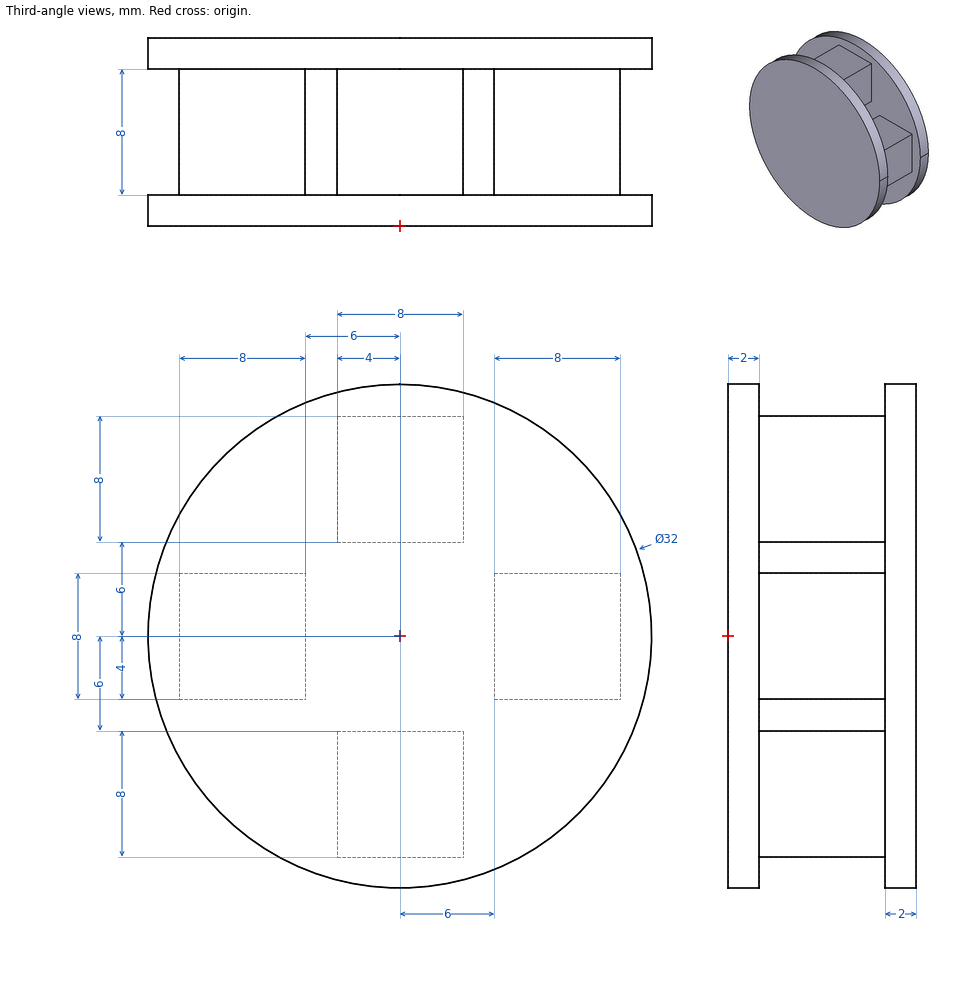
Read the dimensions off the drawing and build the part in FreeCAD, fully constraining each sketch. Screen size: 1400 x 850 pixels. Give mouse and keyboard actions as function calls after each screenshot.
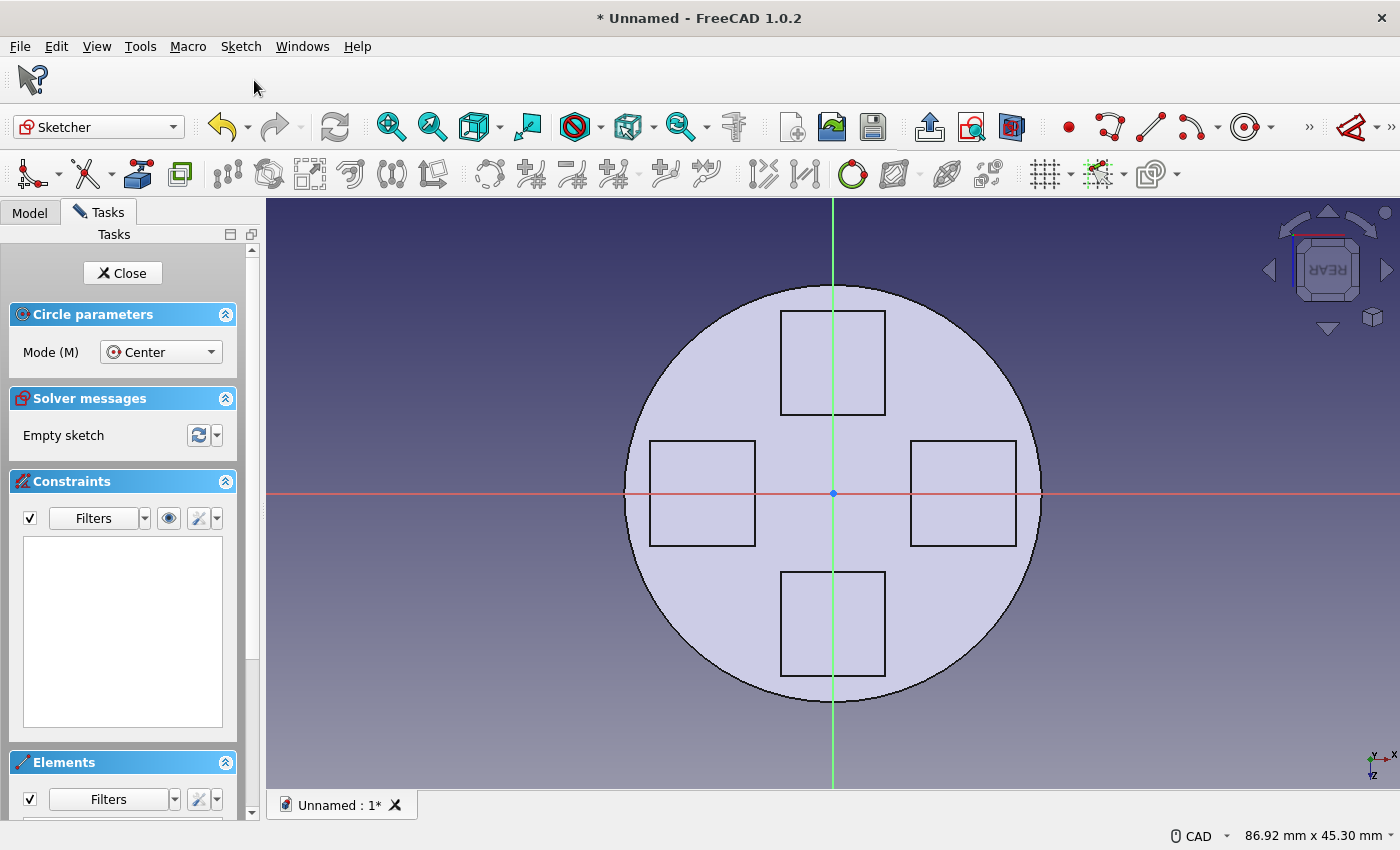
click(833, 493)
click(981, 346)
key(Escape)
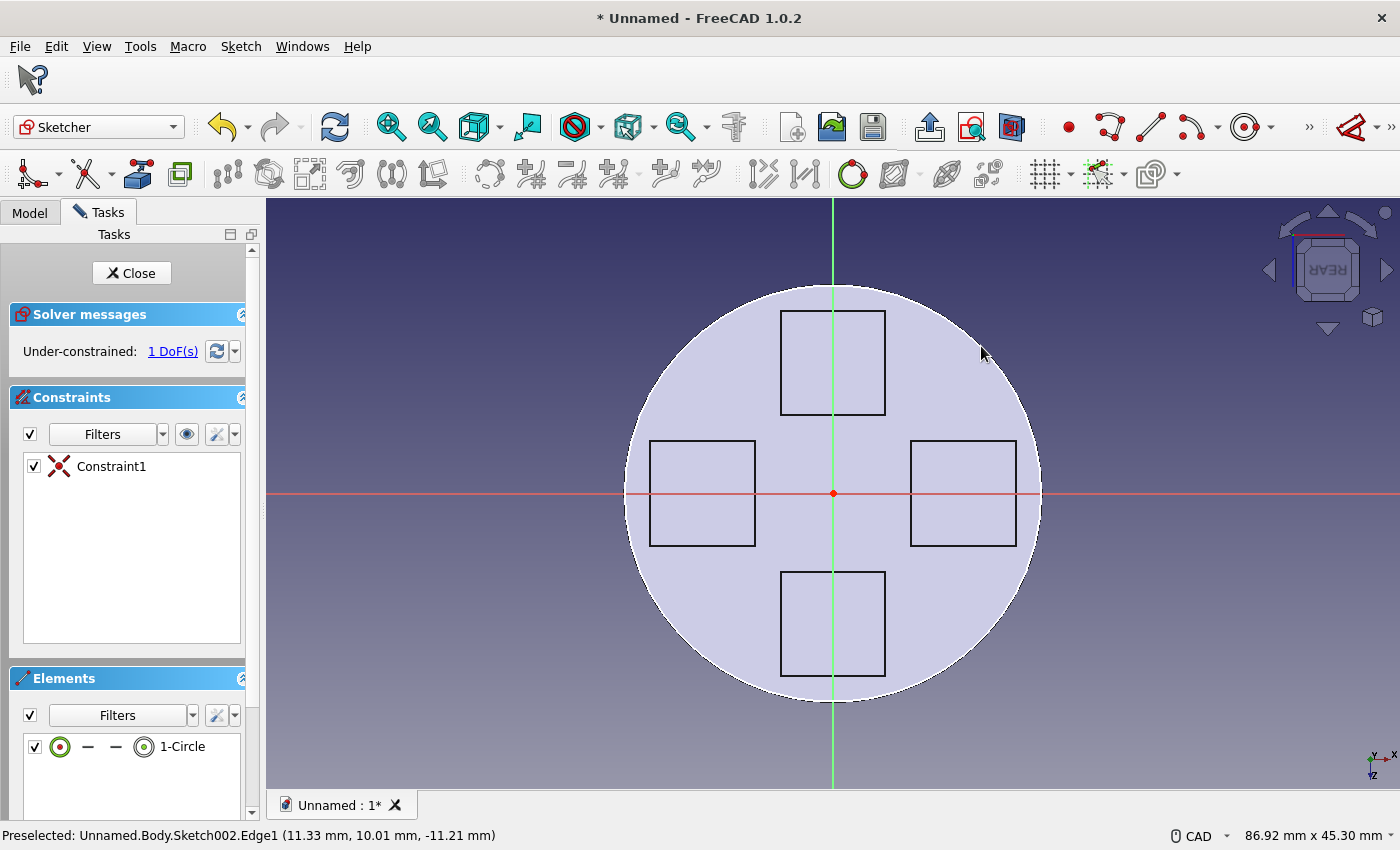
click(1350, 128)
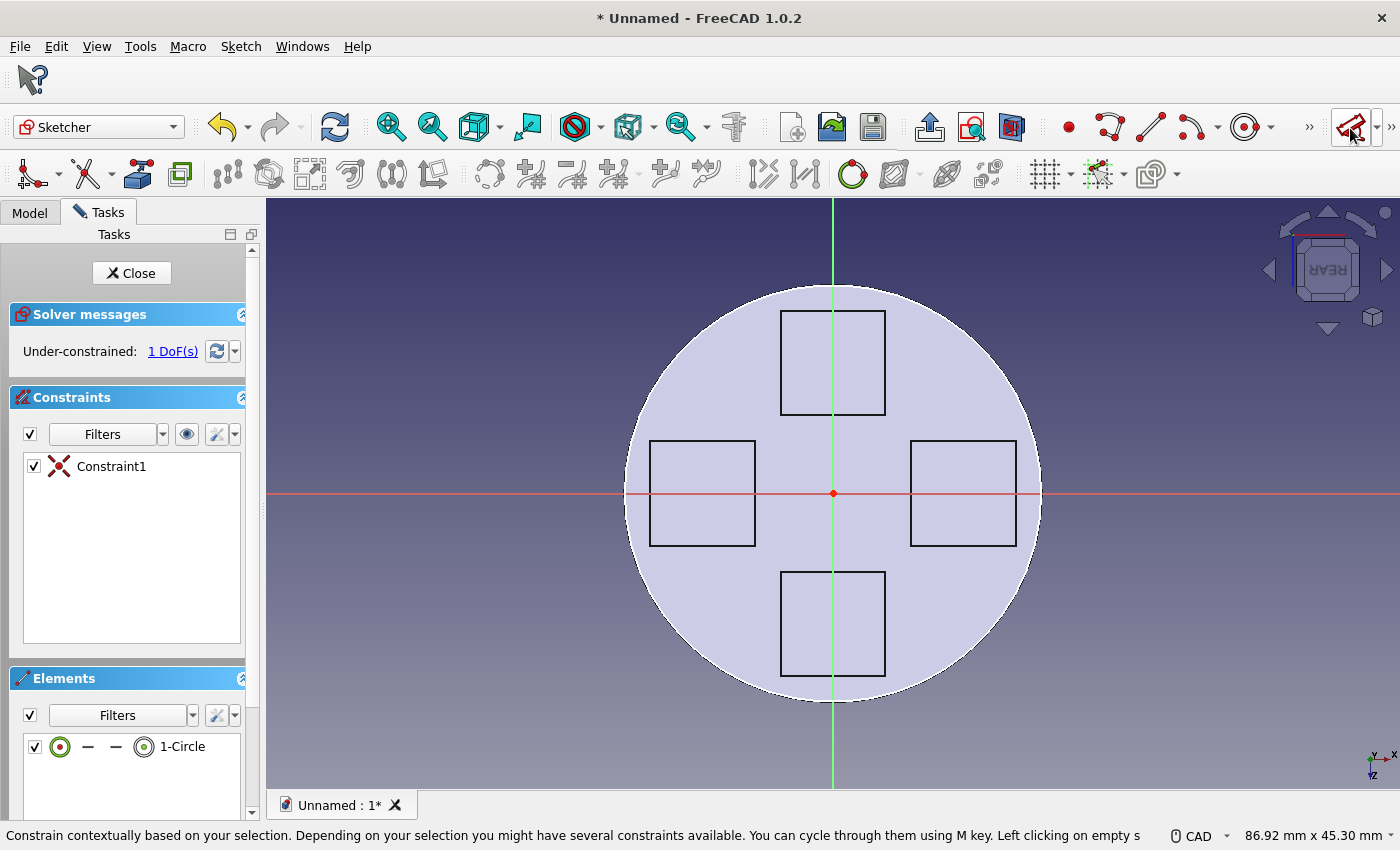
click(980, 346)
click(1003, 323)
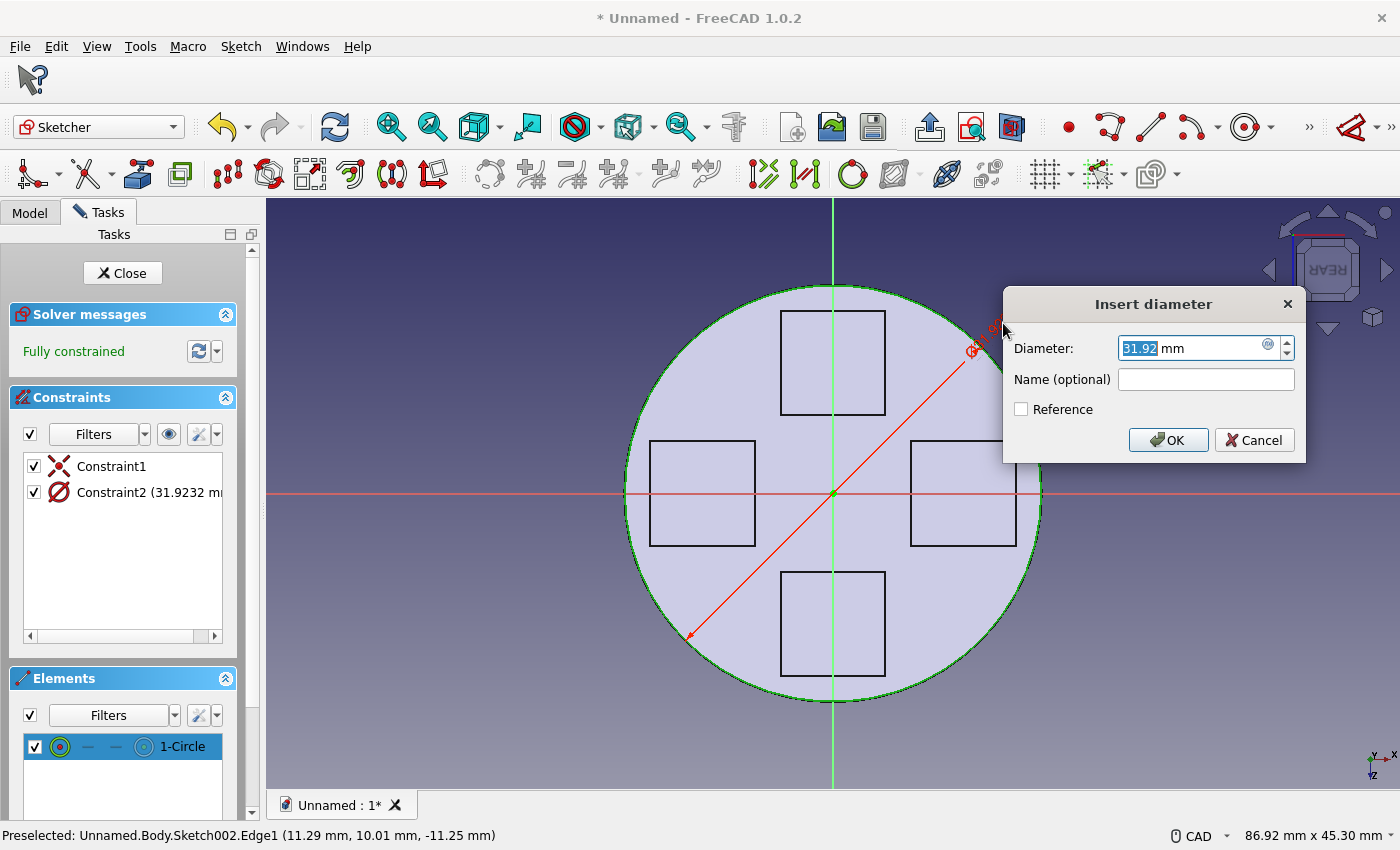
text(32)
key(Return)
key(Escape)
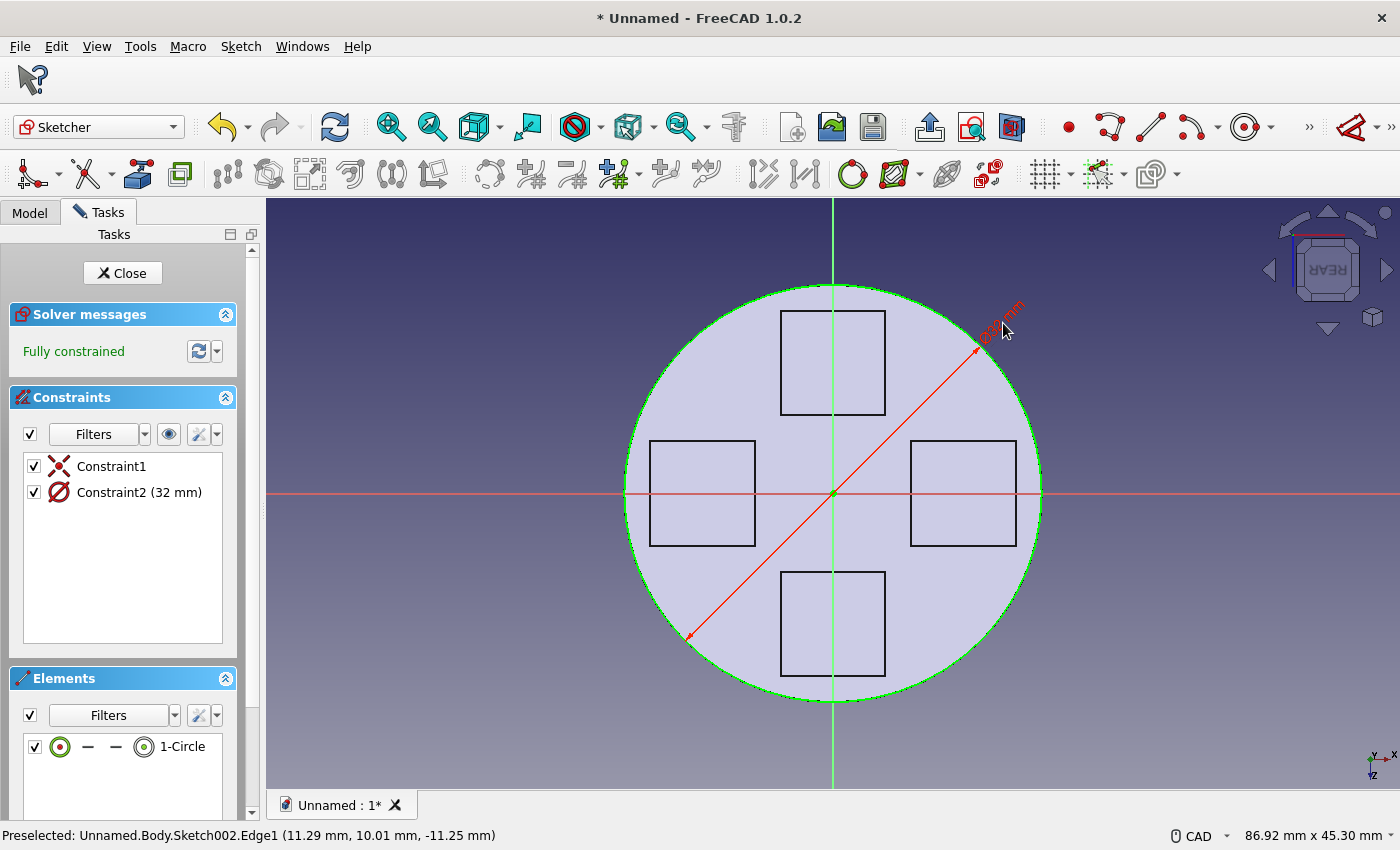
click(123, 273)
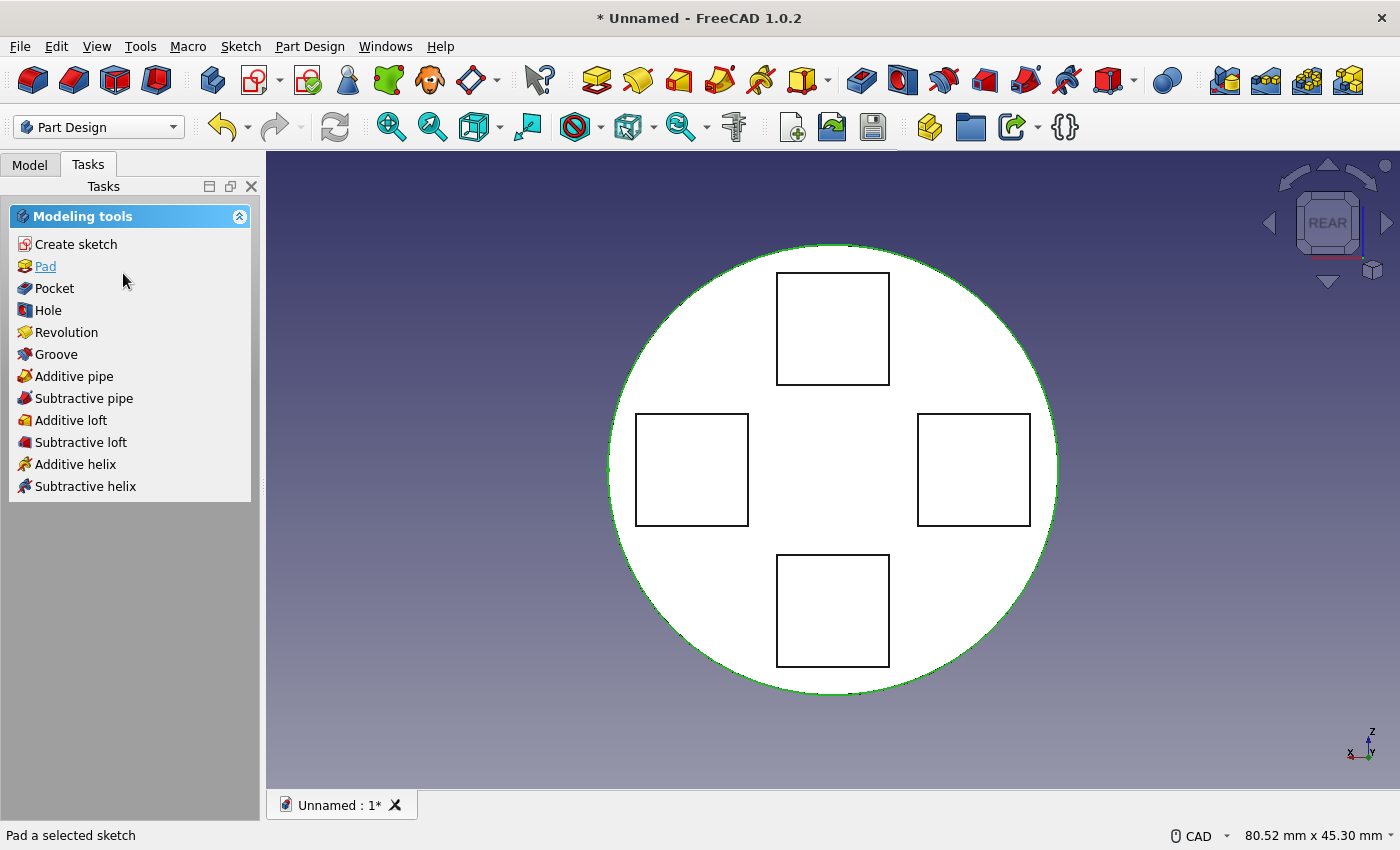
click(597, 80)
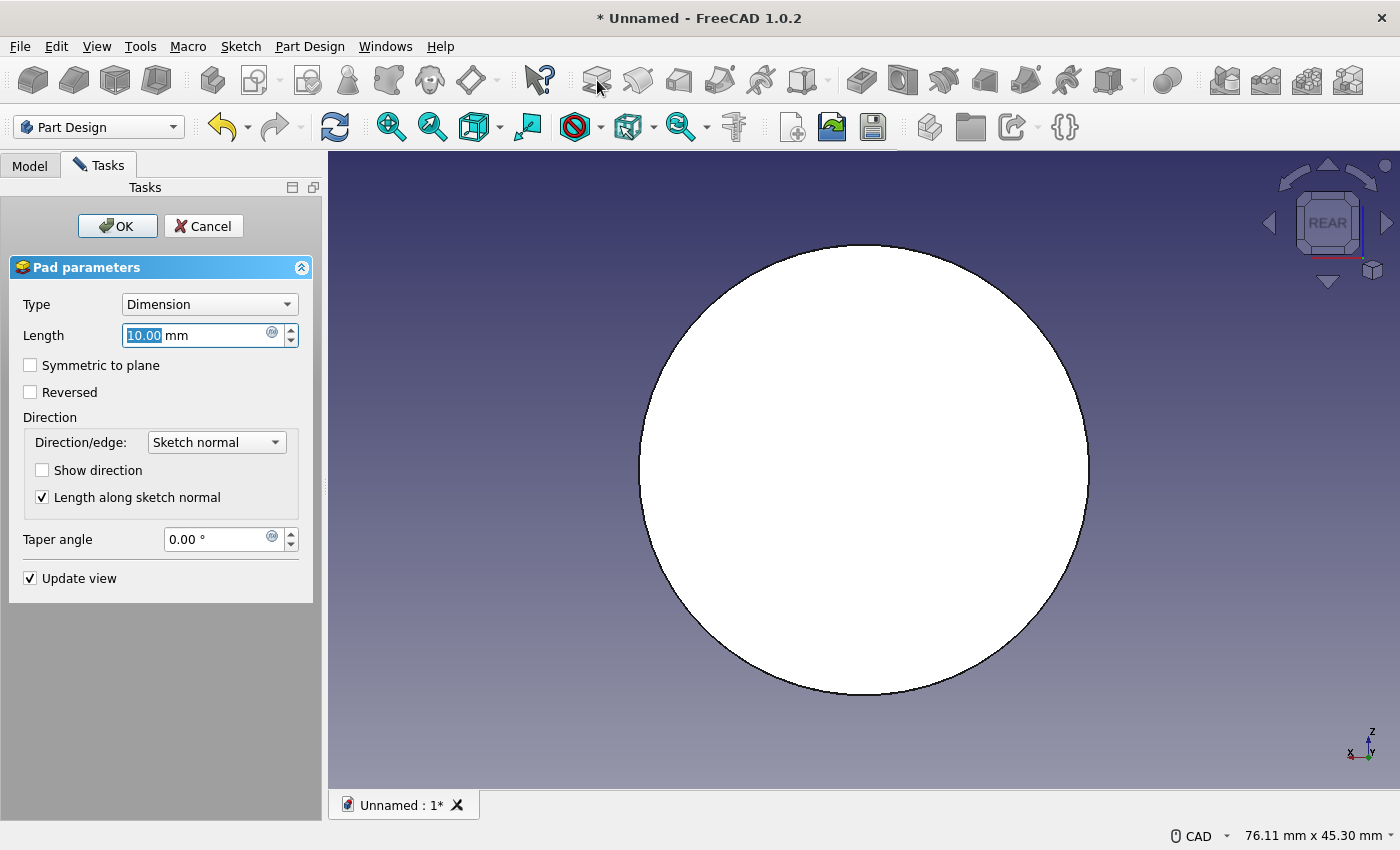
text(2)
key(Tab)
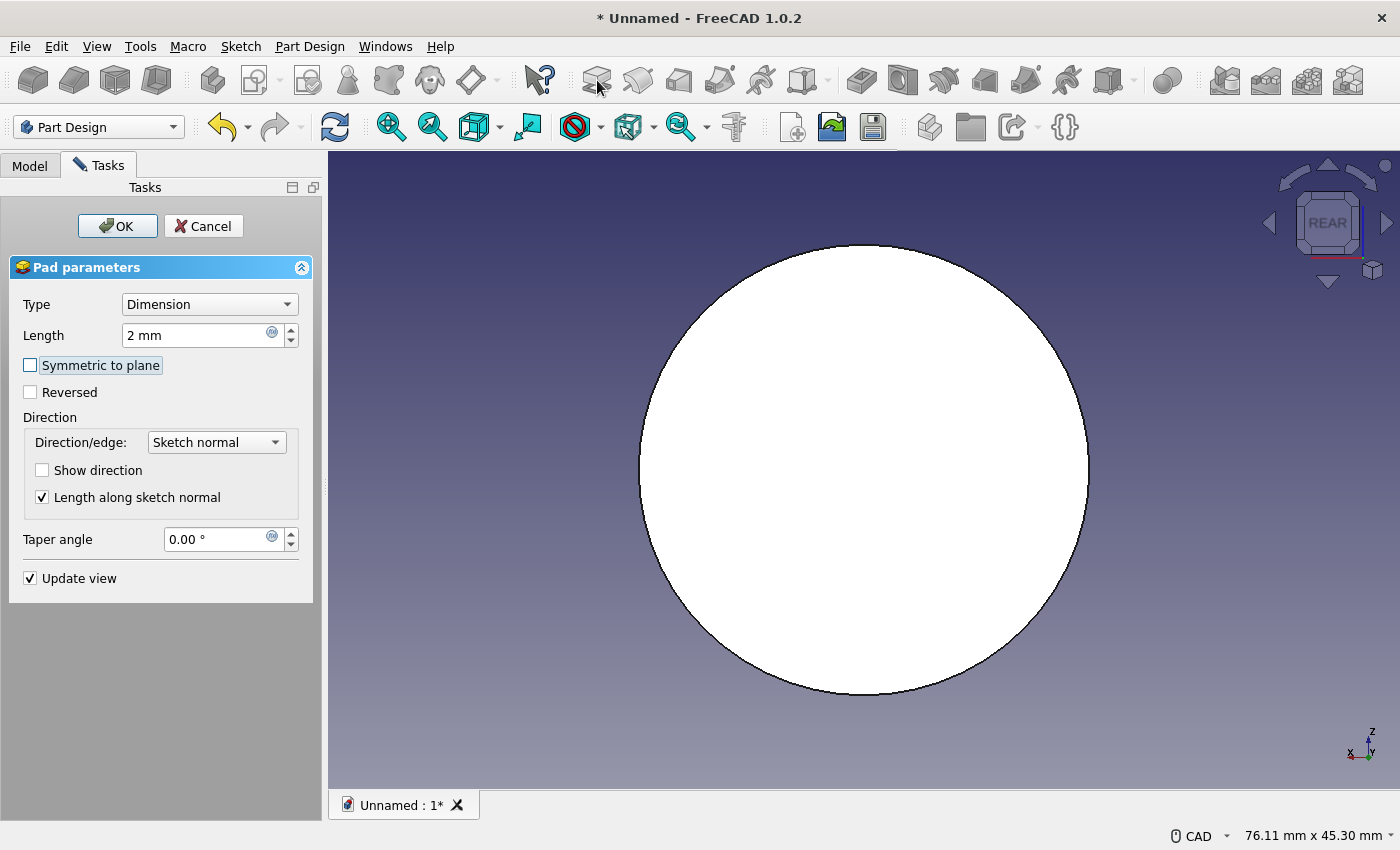
click(118, 226)